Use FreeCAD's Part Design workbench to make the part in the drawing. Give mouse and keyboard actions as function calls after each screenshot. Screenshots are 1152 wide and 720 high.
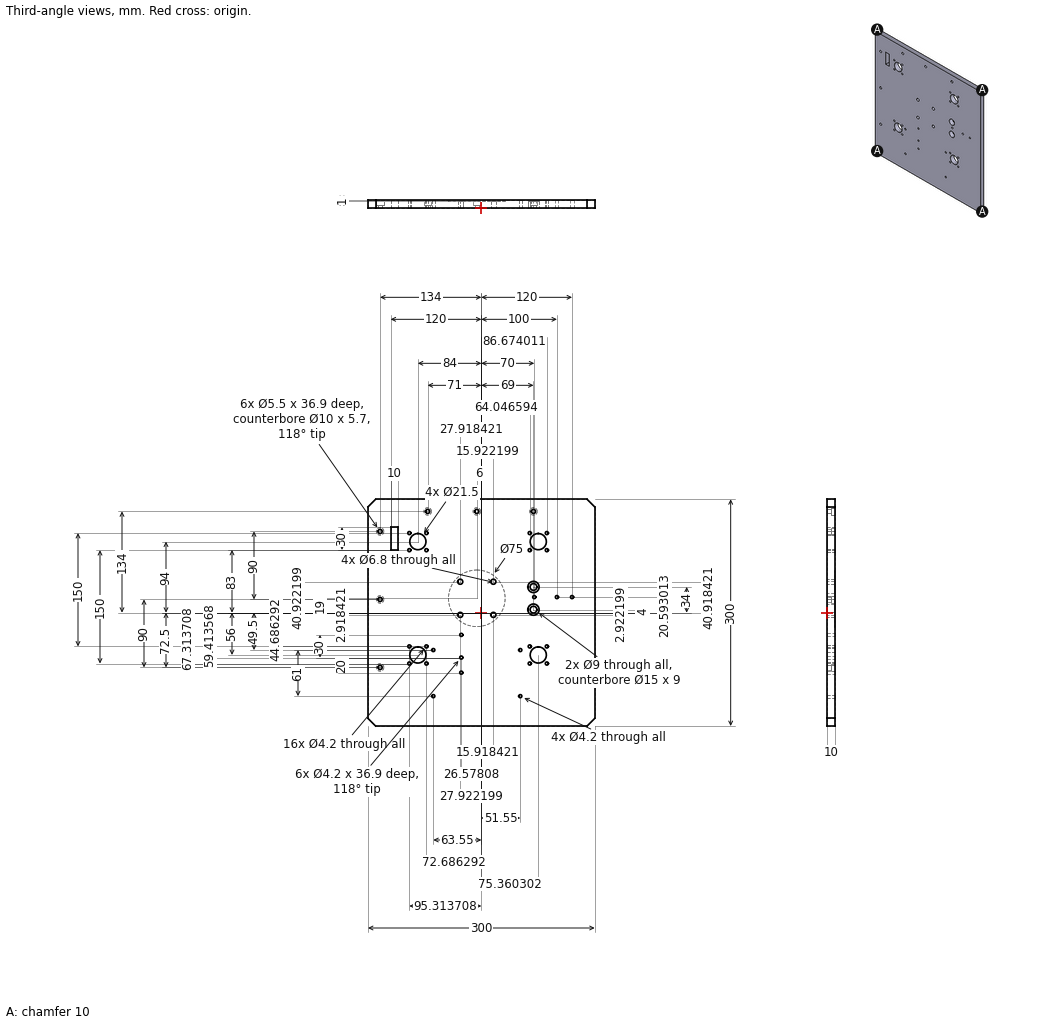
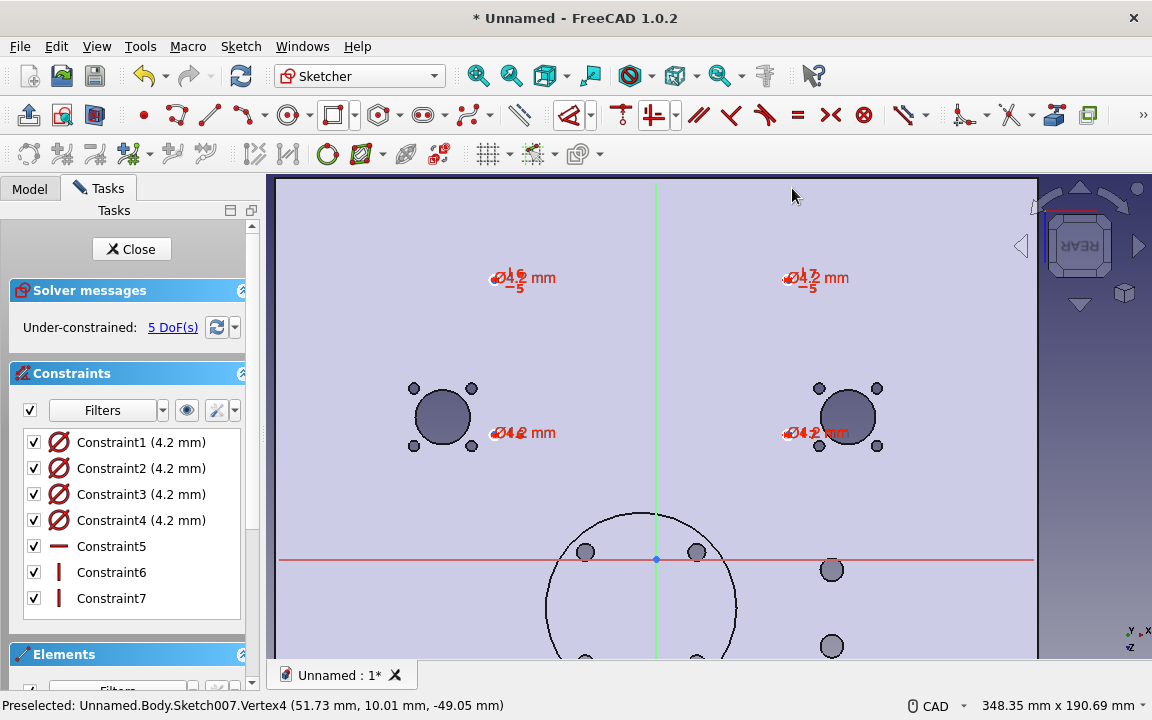
click(495, 435)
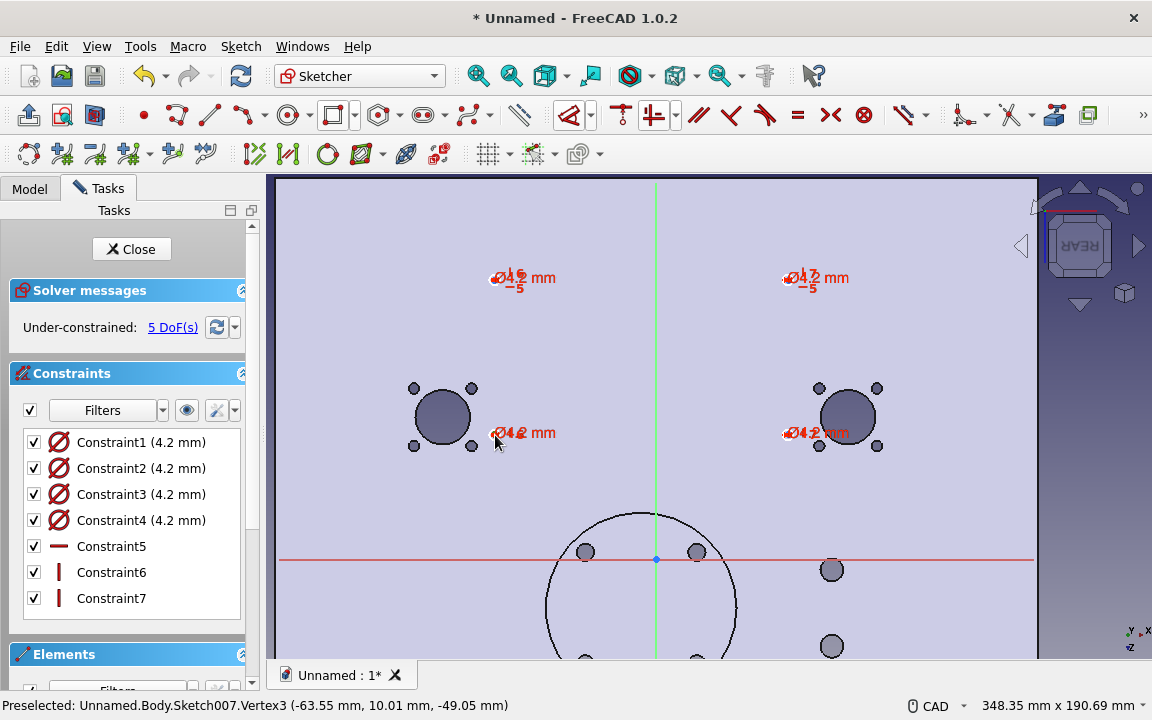
click(788, 435)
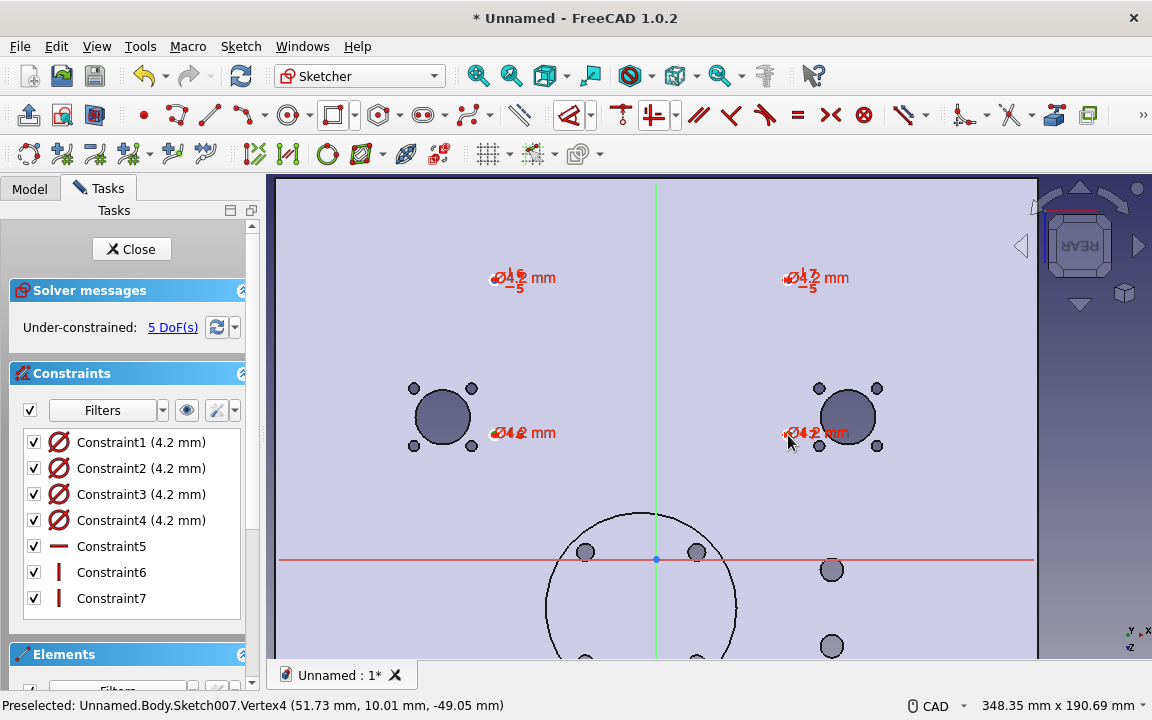
click(676, 116)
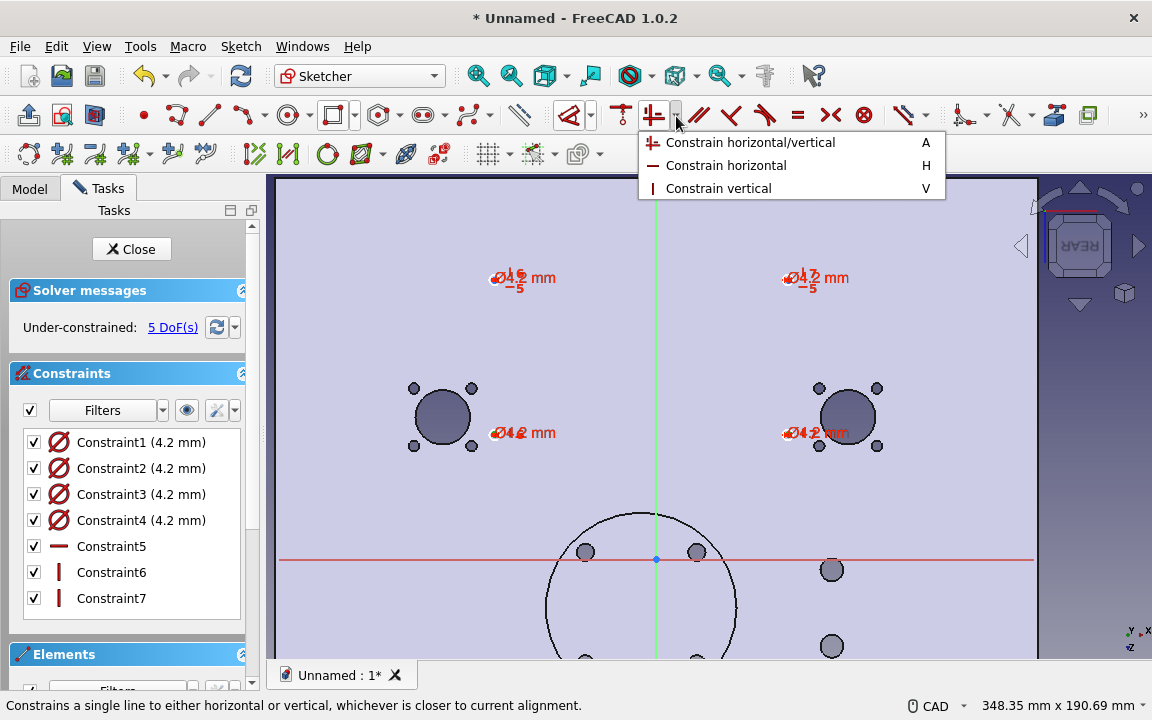
click(792, 166)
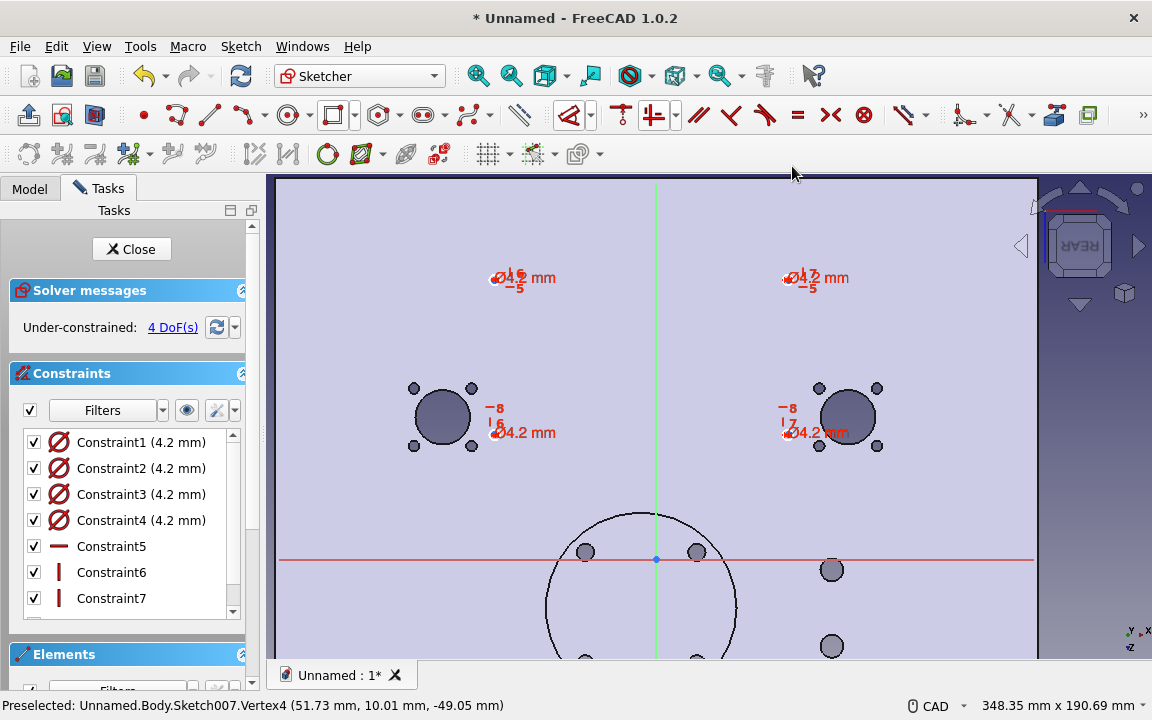
click(495, 280)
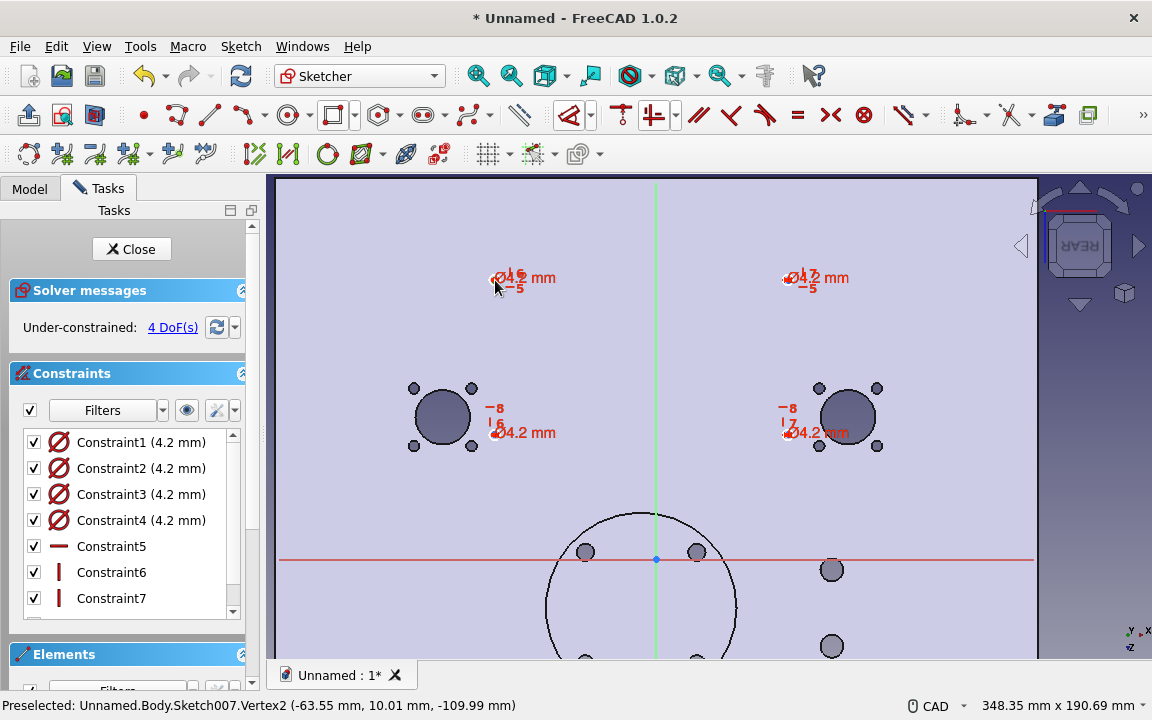
click(495, 435)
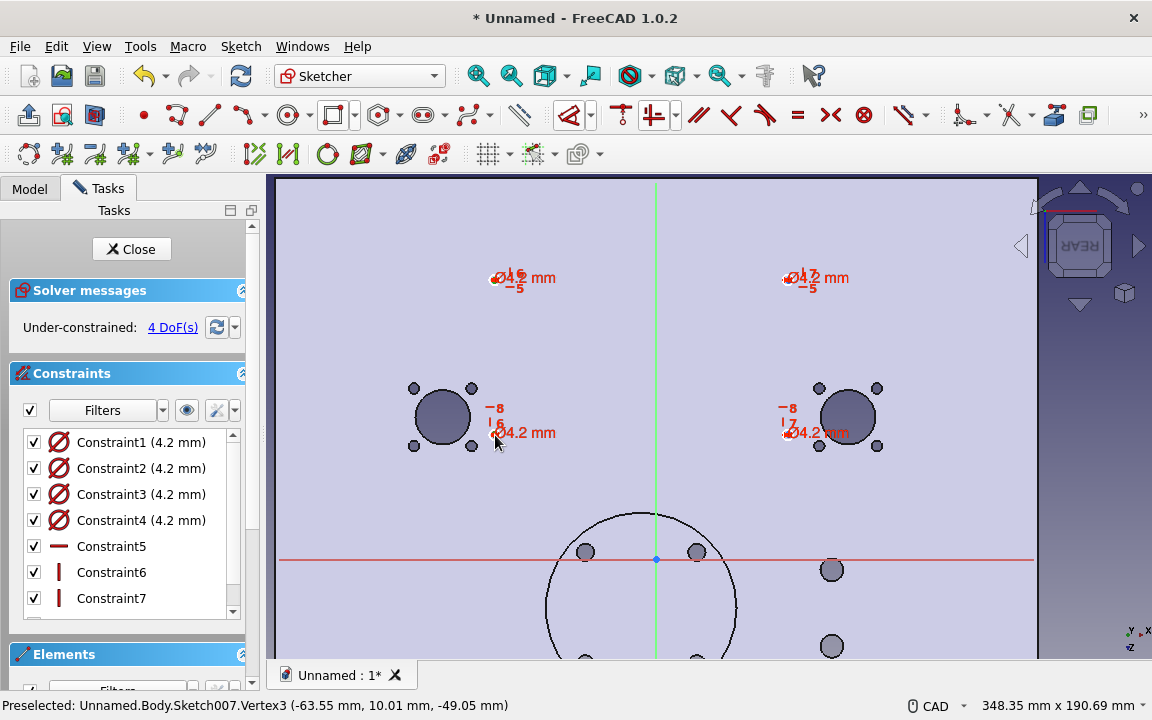
key(i)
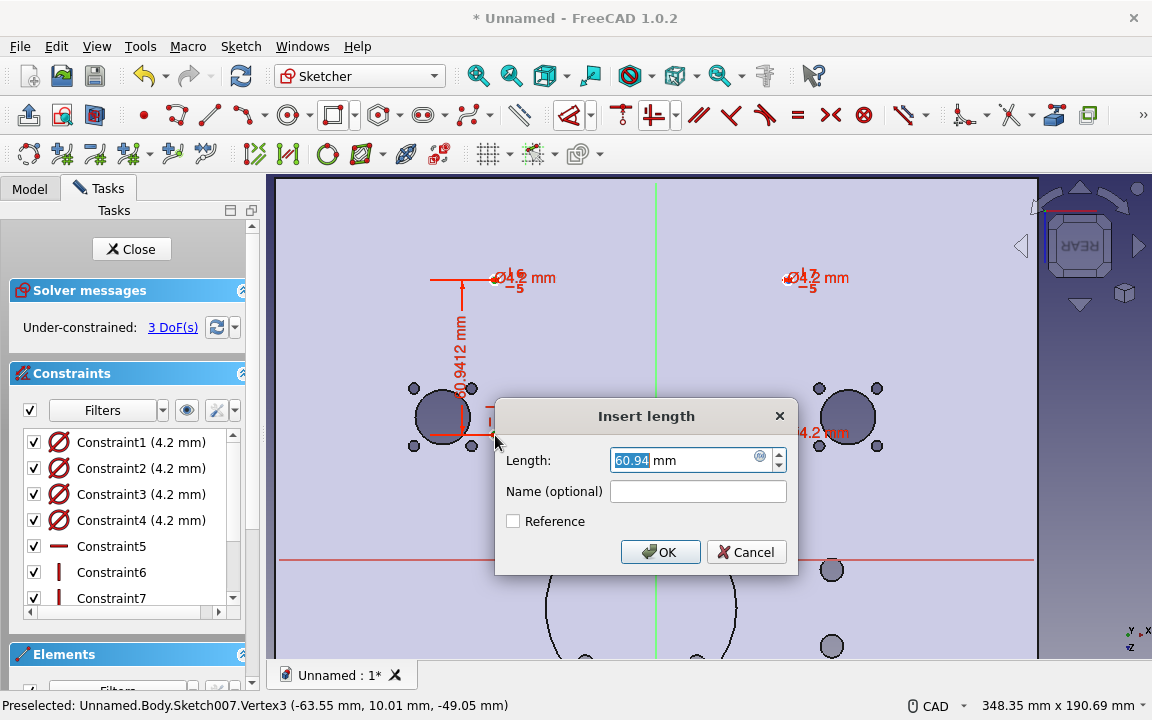
text(61)
key(Return)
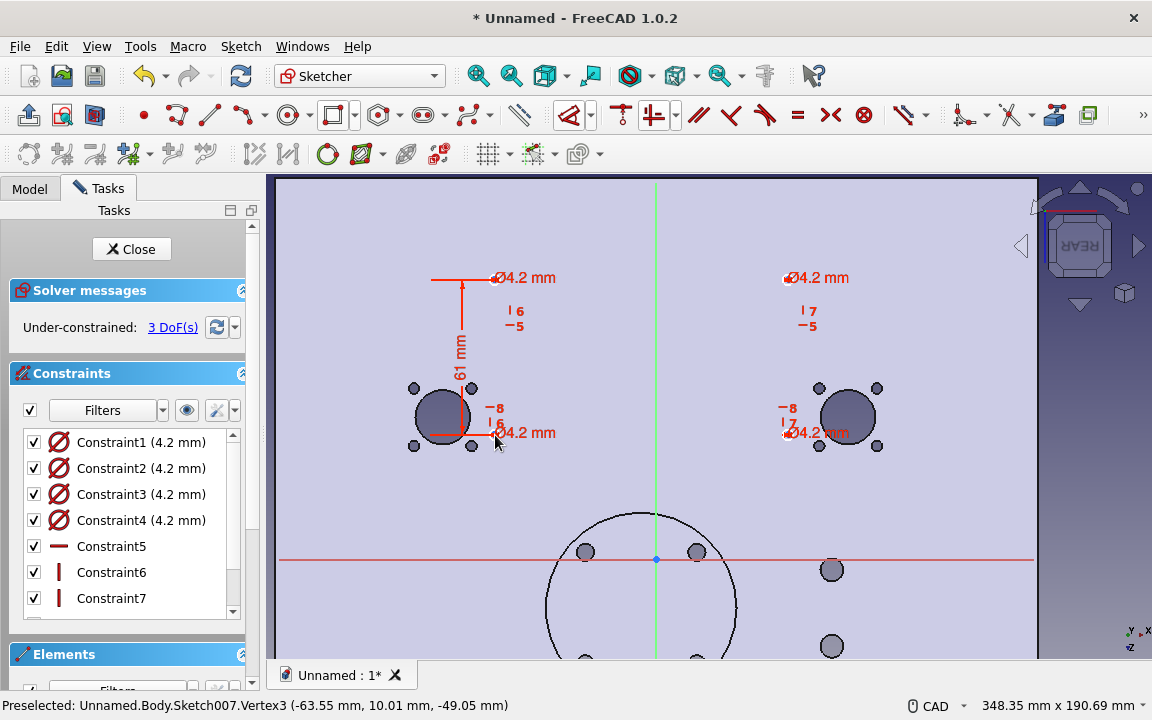
click(495, 435)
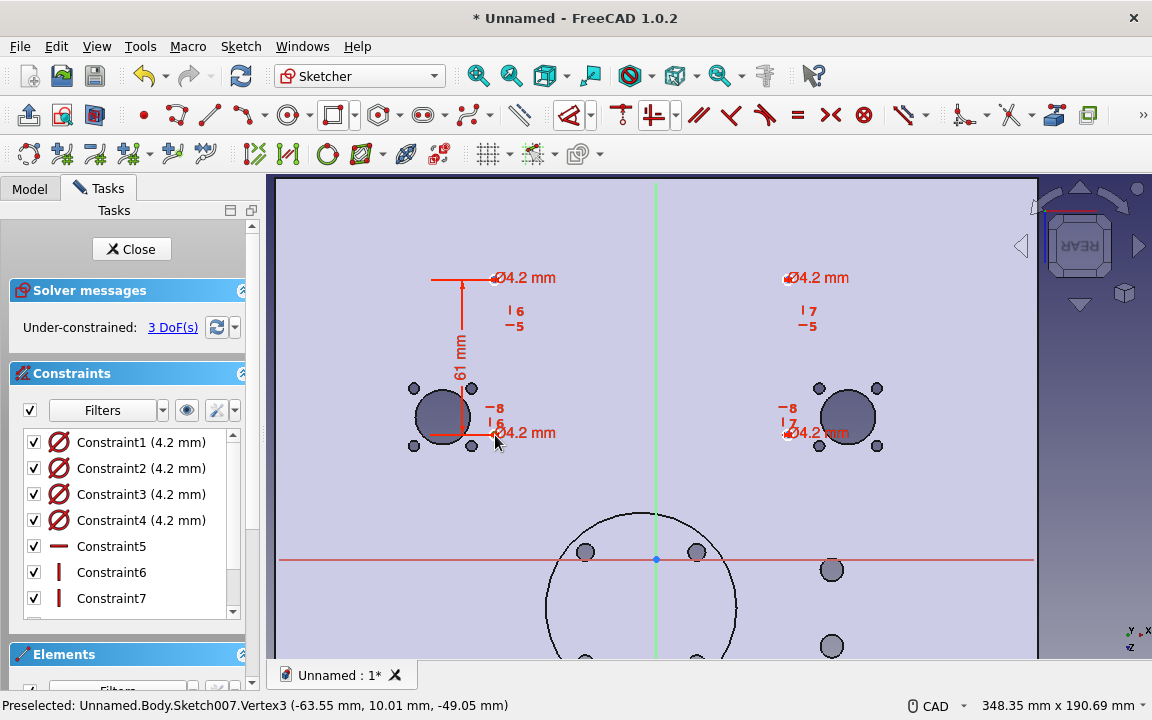
click(590, 116)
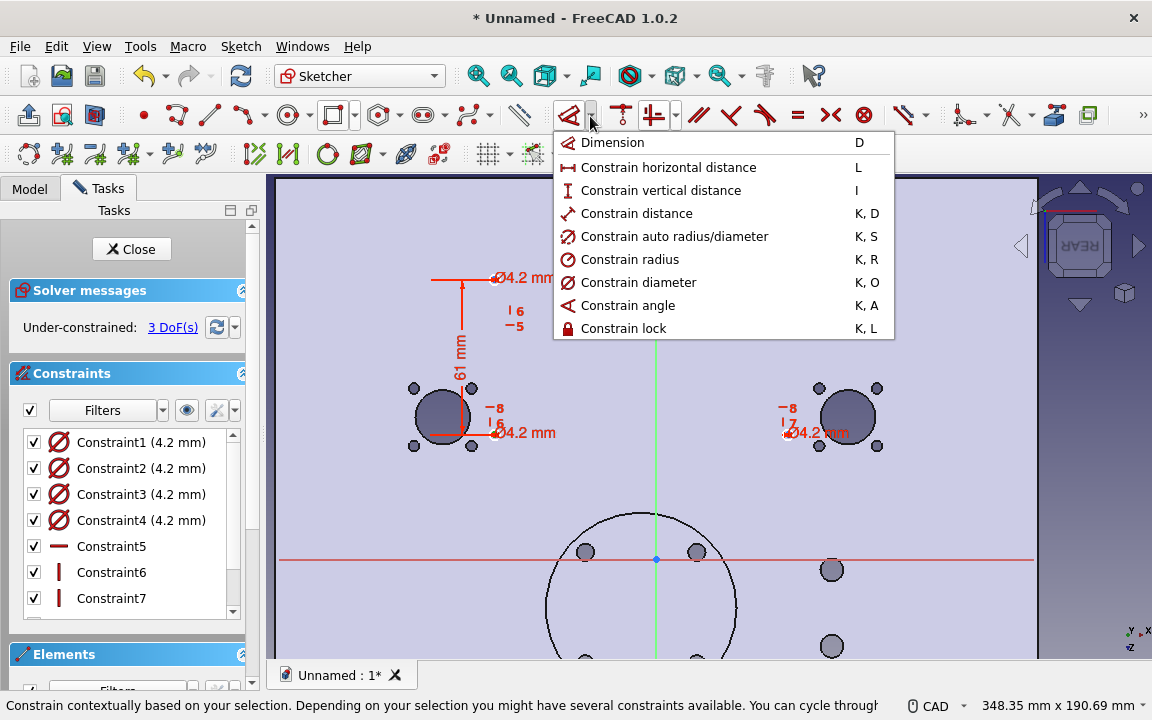
click(724, 190)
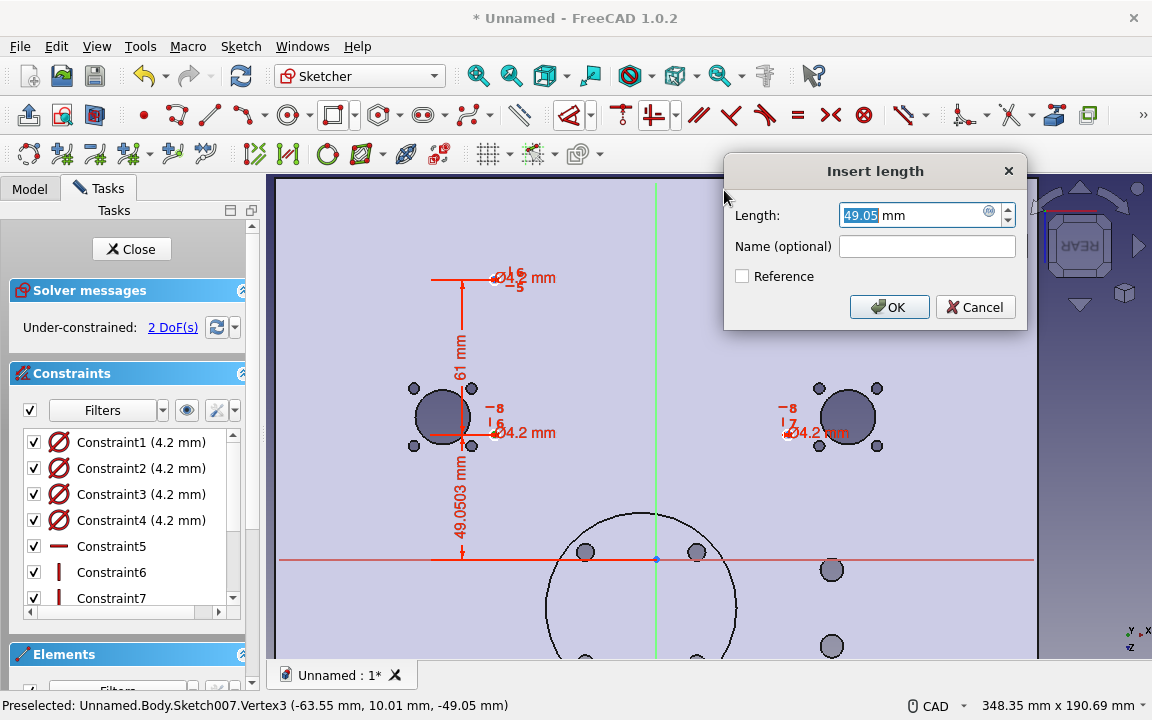
text(49.5)
key(Return)